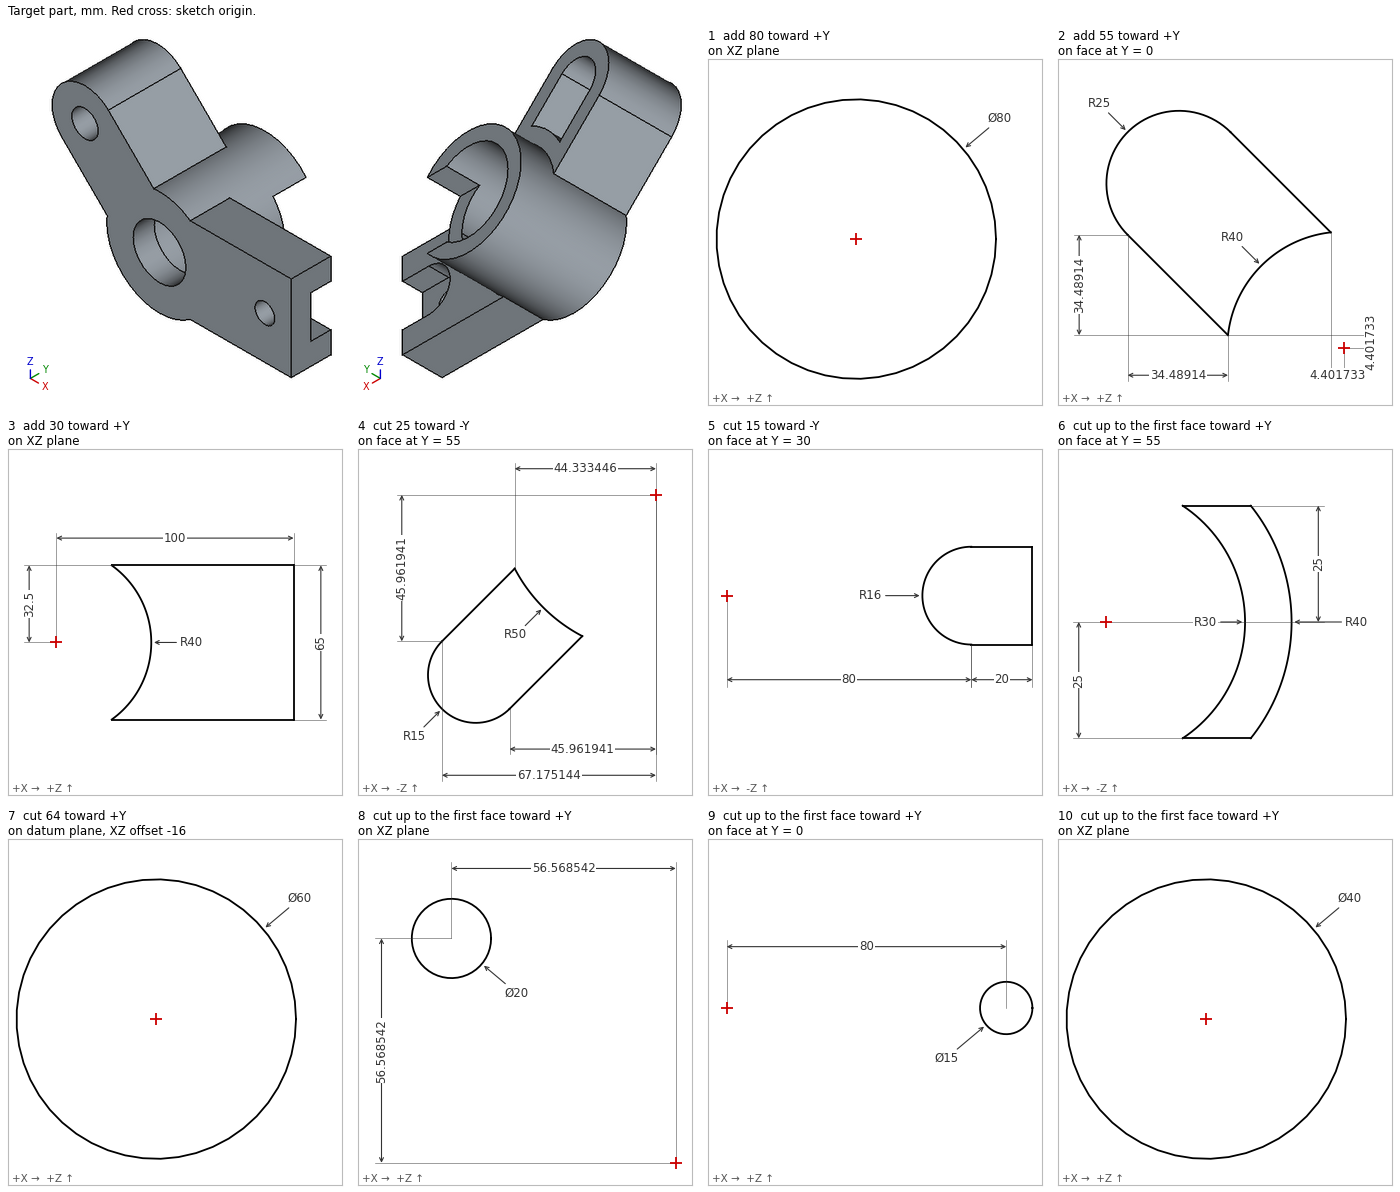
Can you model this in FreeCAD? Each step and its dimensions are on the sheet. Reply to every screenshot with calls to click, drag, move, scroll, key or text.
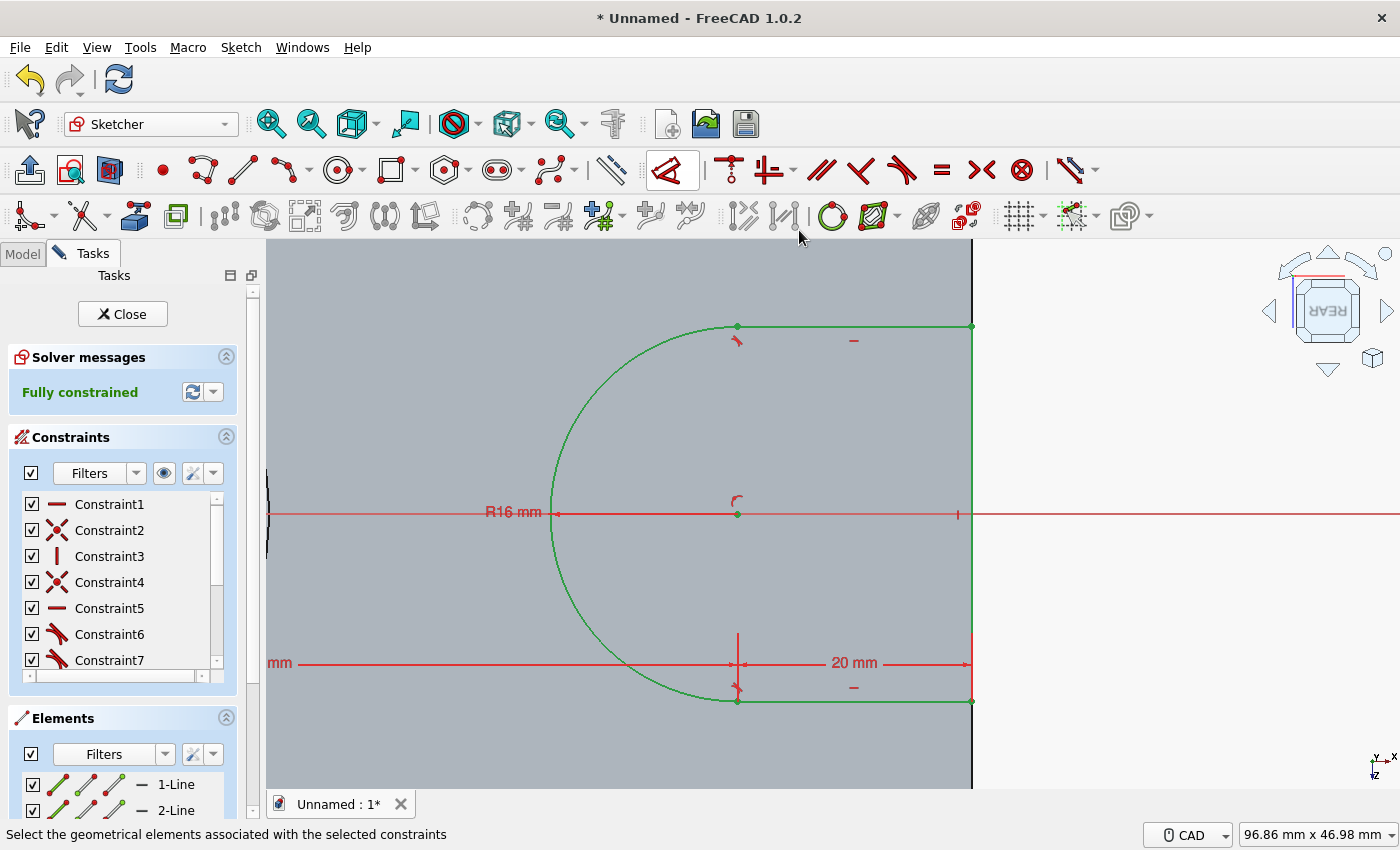
click(123, 314)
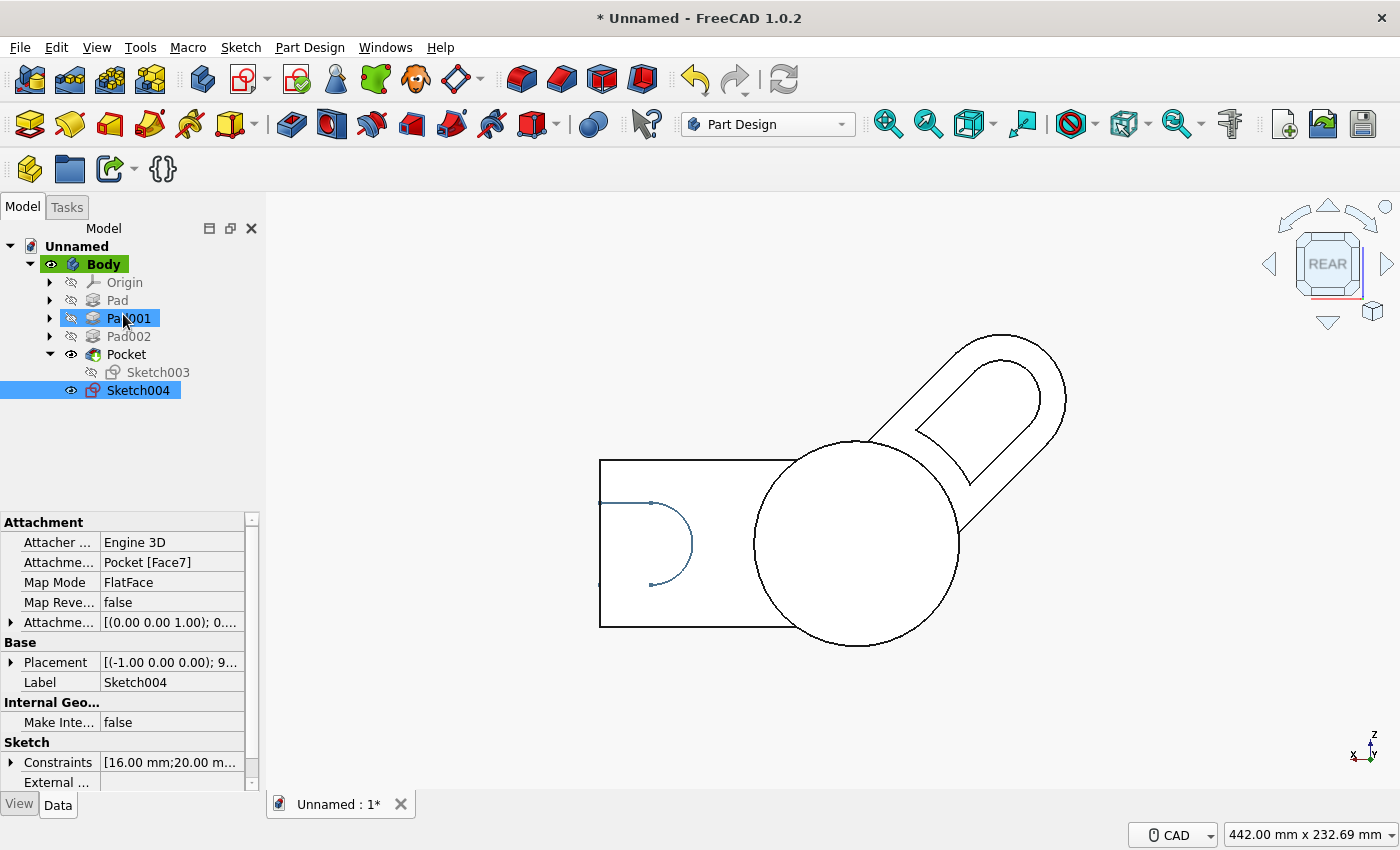
click(292, 124)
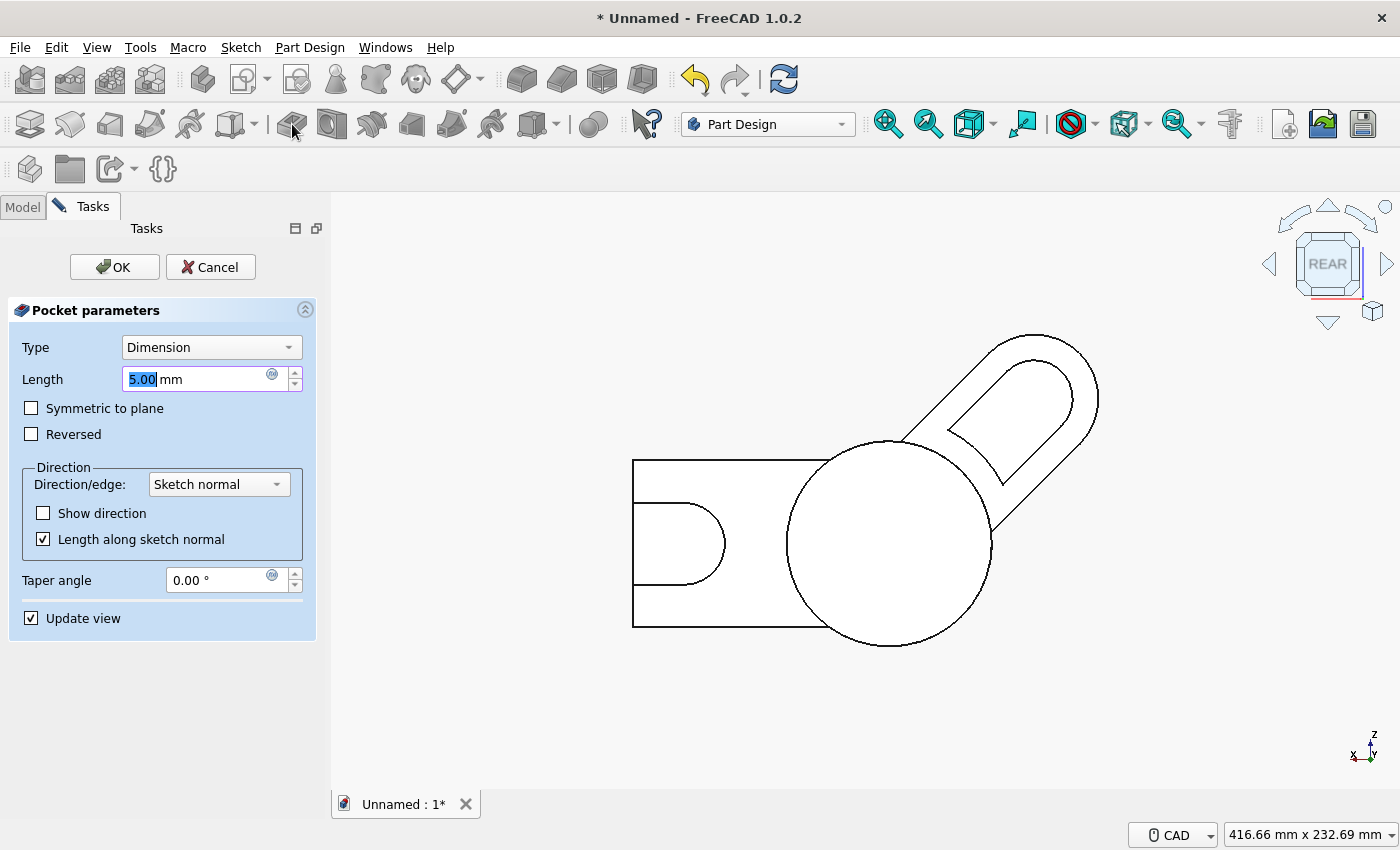
text(15)
key(Tab)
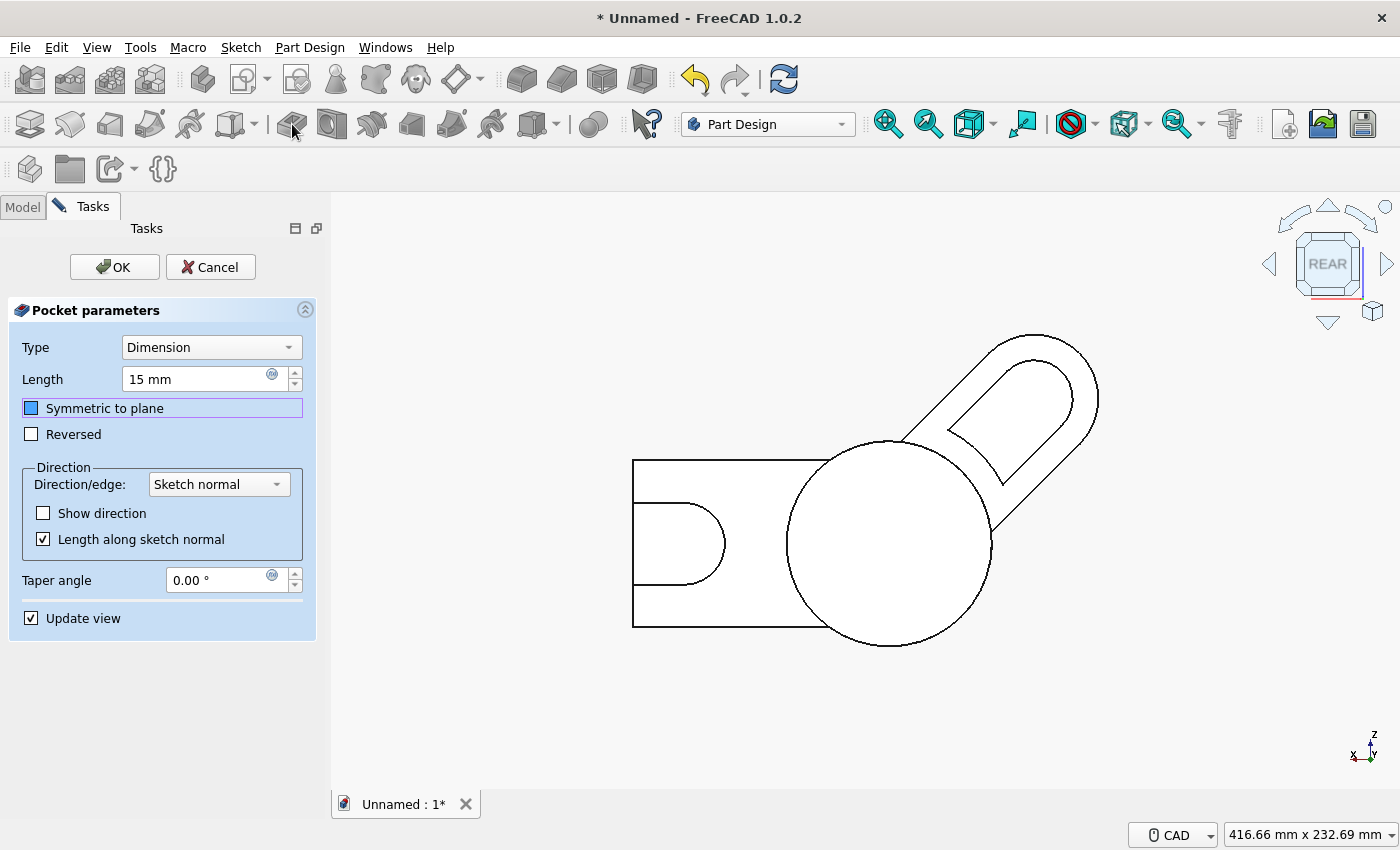
click(115, 267)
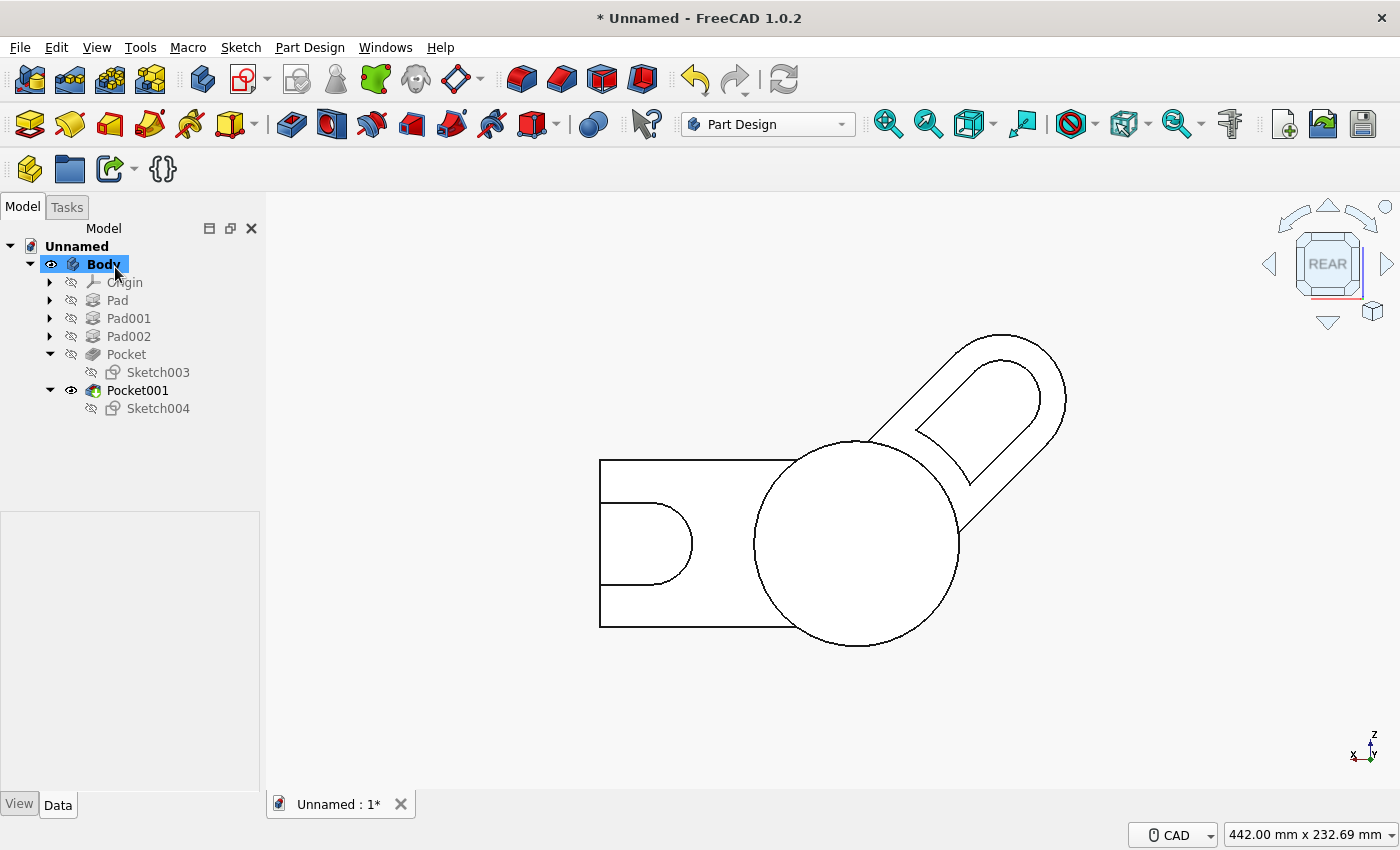
click(939, 461)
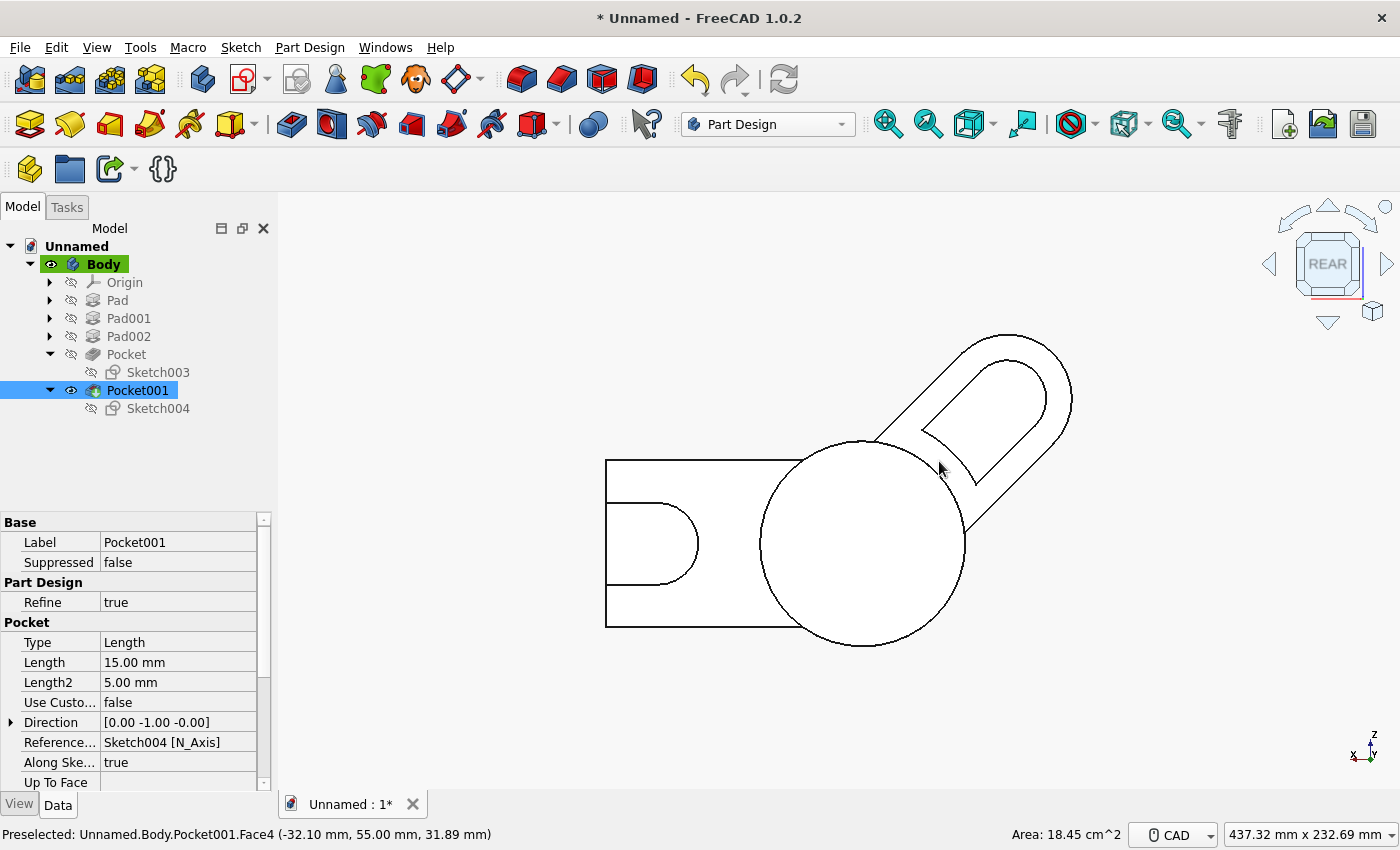
click(244, 80)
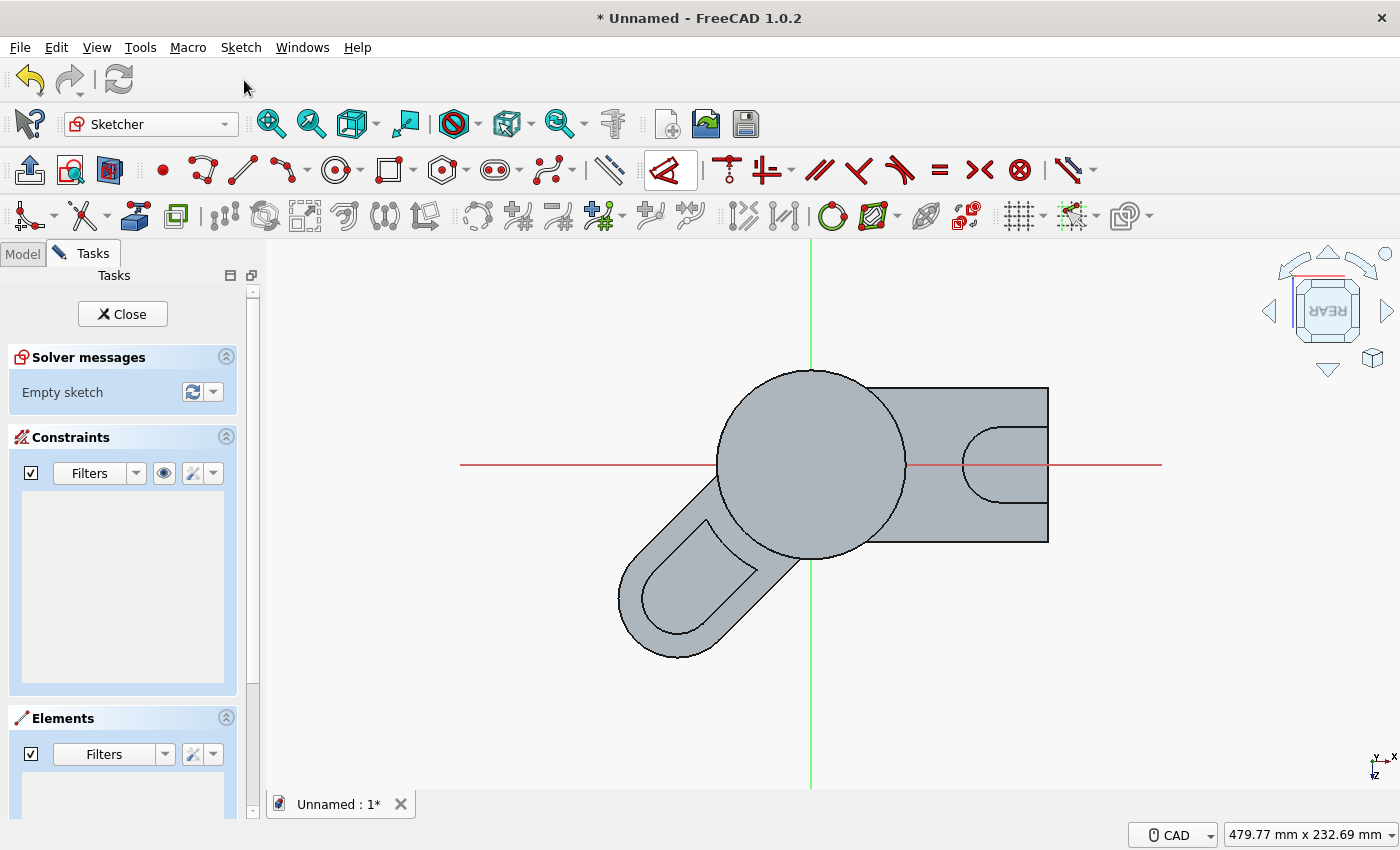
click(110, 170)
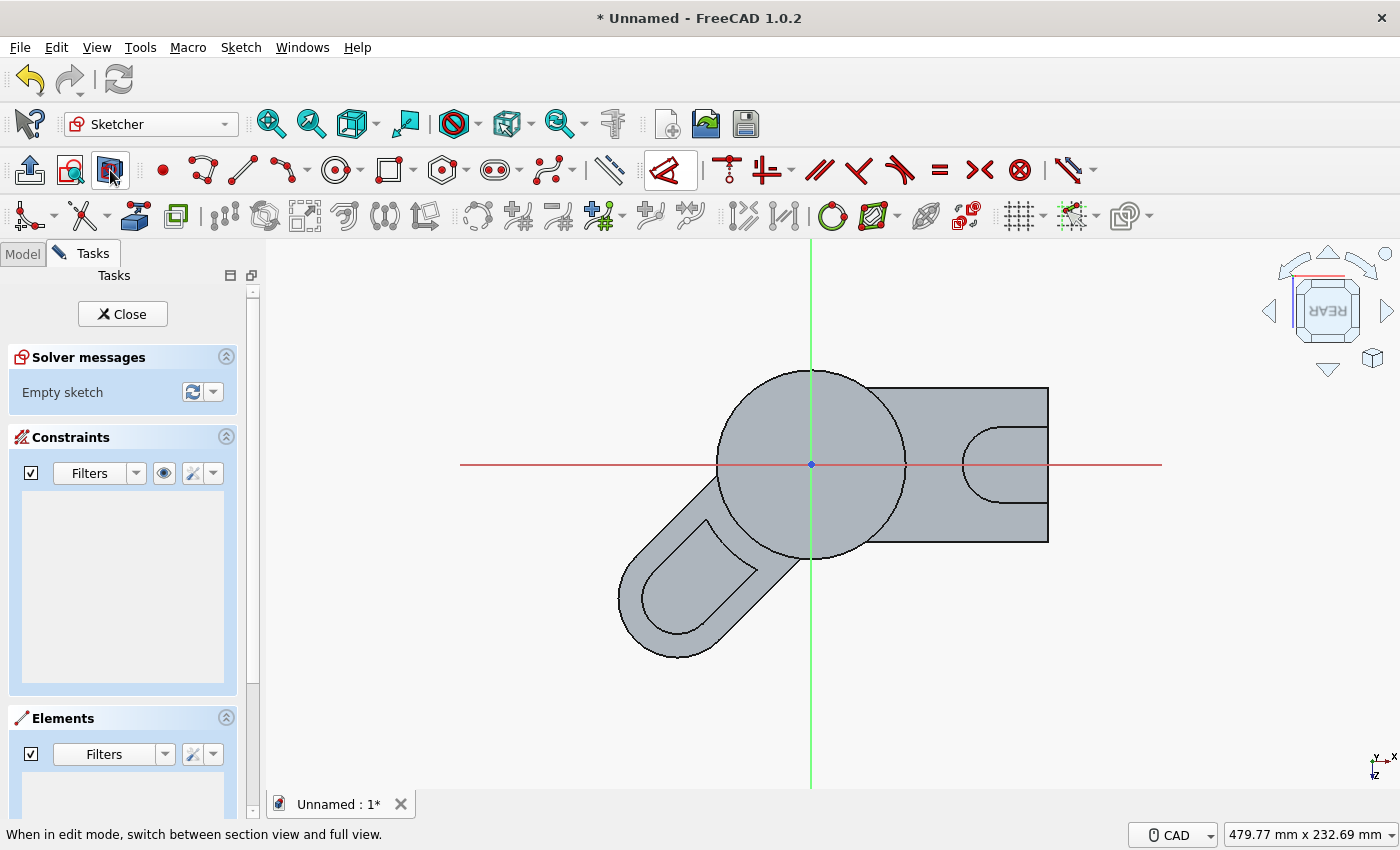
scroll(913, 436, up, 5)